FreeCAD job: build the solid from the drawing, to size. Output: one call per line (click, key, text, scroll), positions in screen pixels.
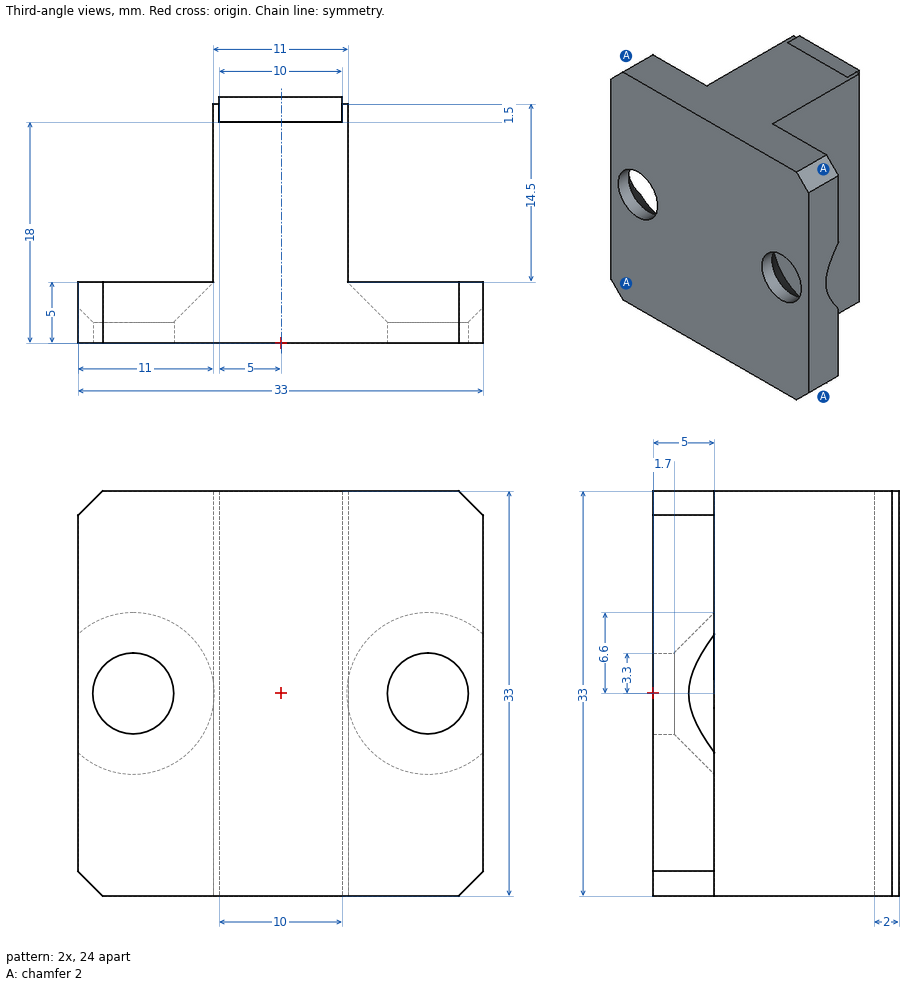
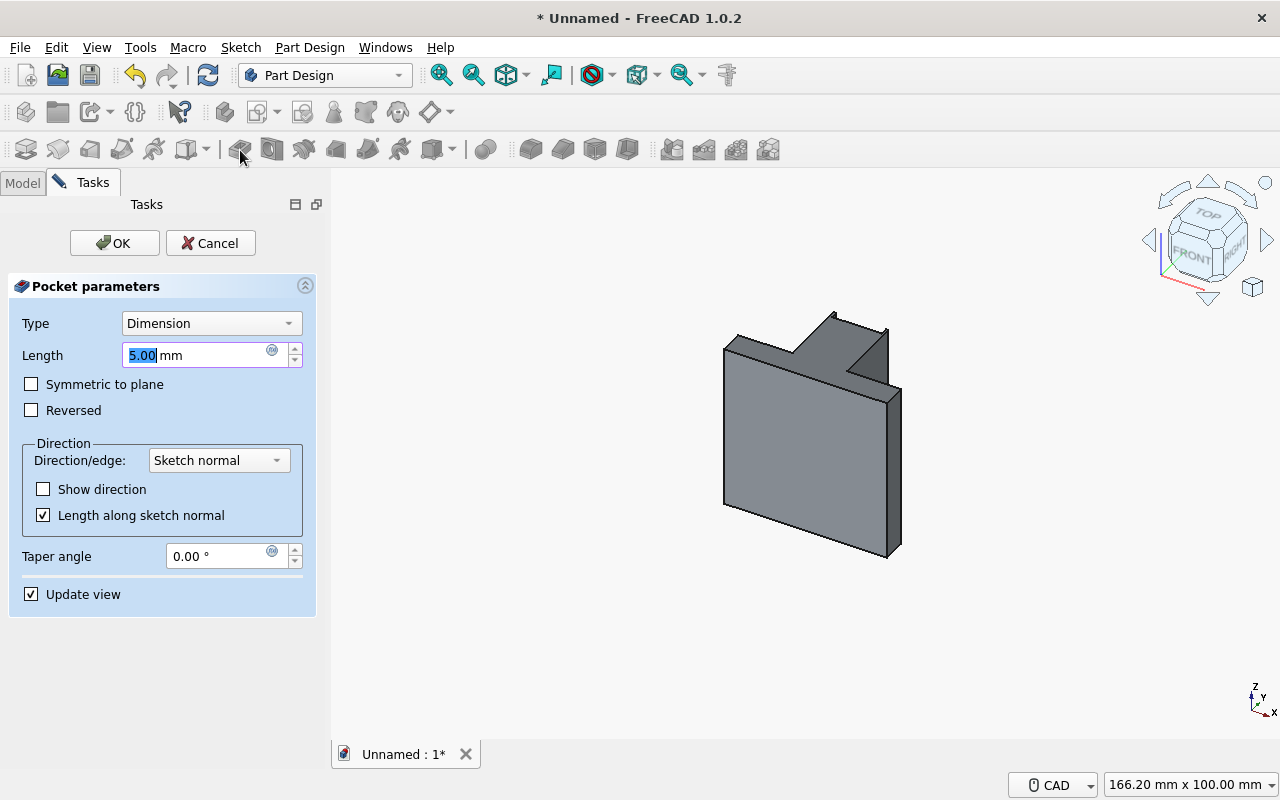
click(212, 324)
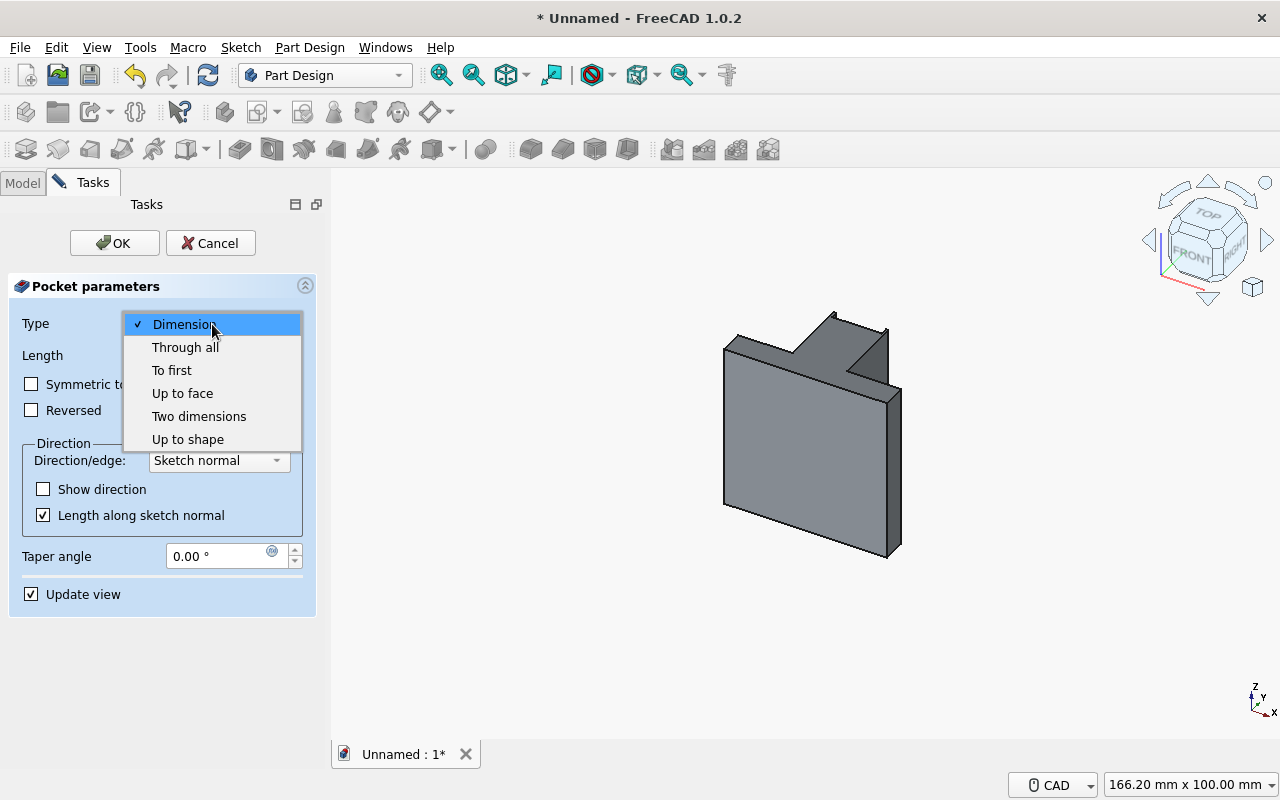
click(212, 348)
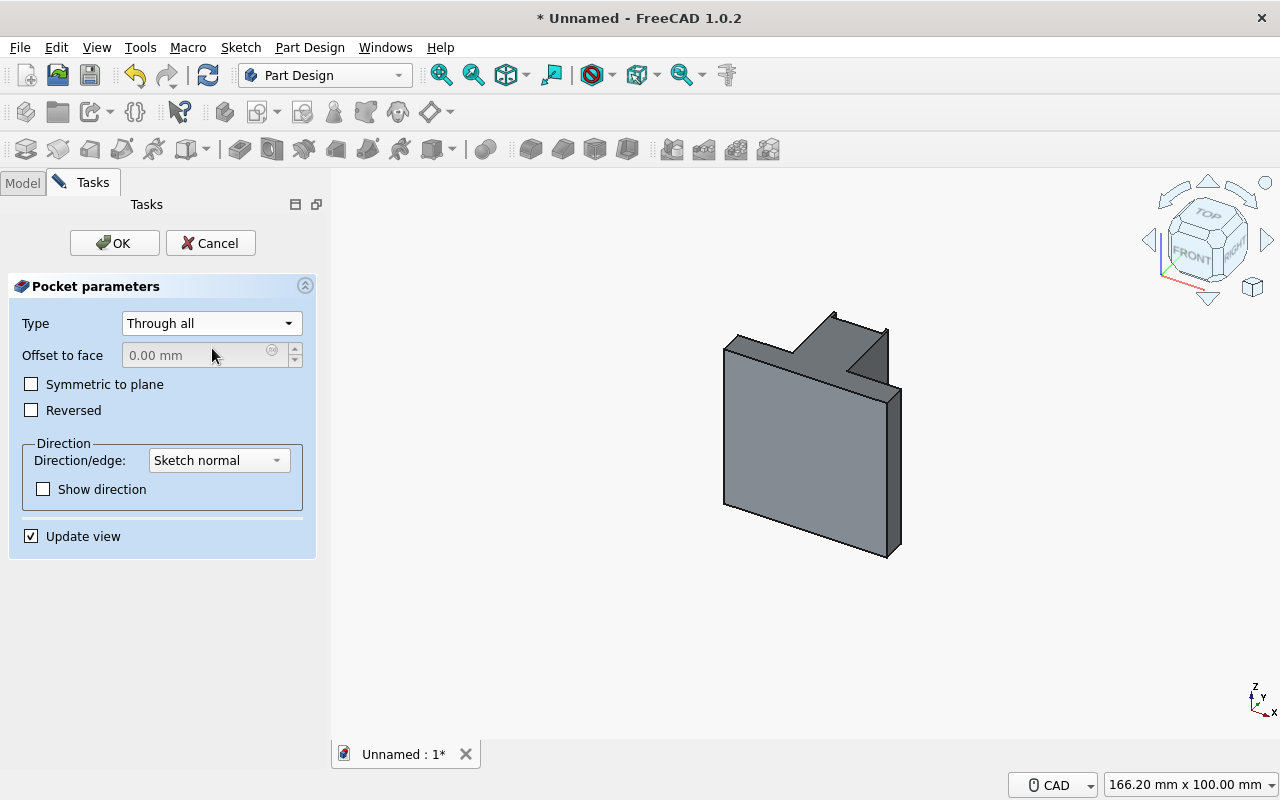
click(115, 243)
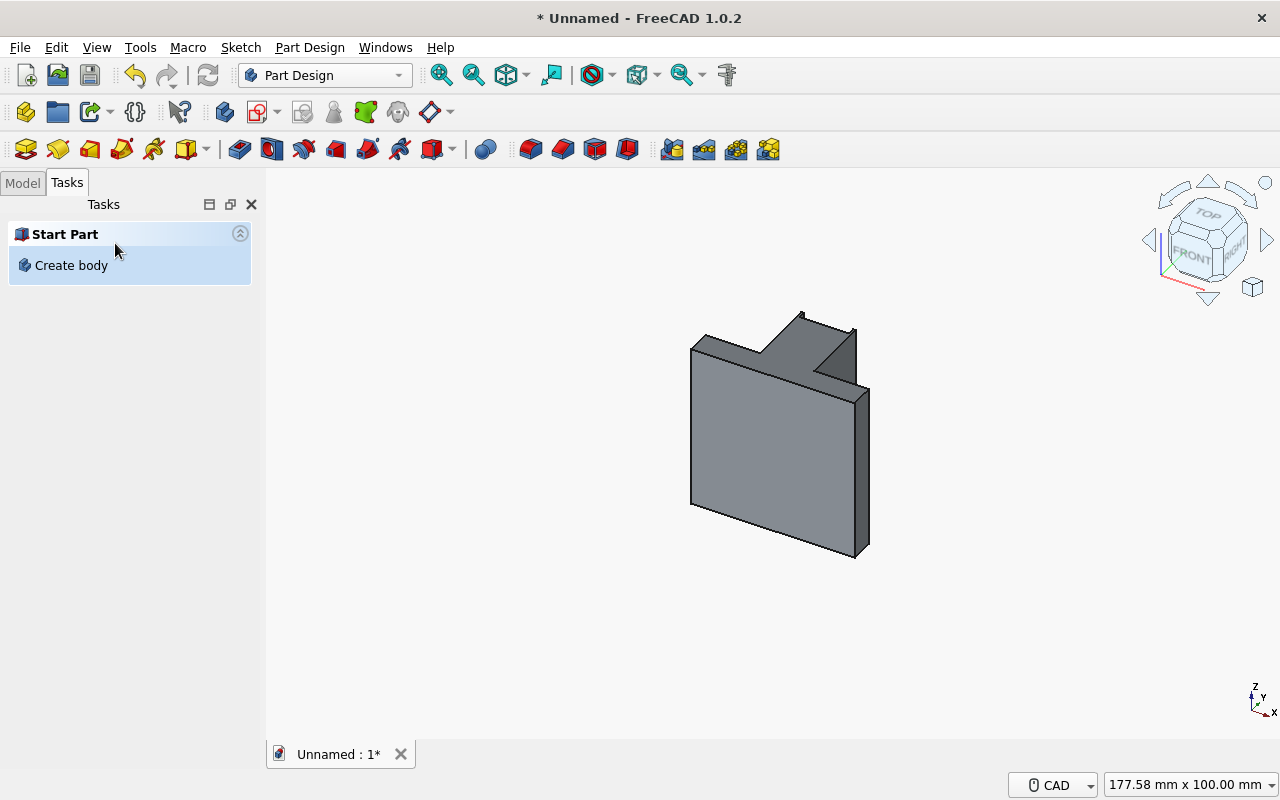
click(23, 182)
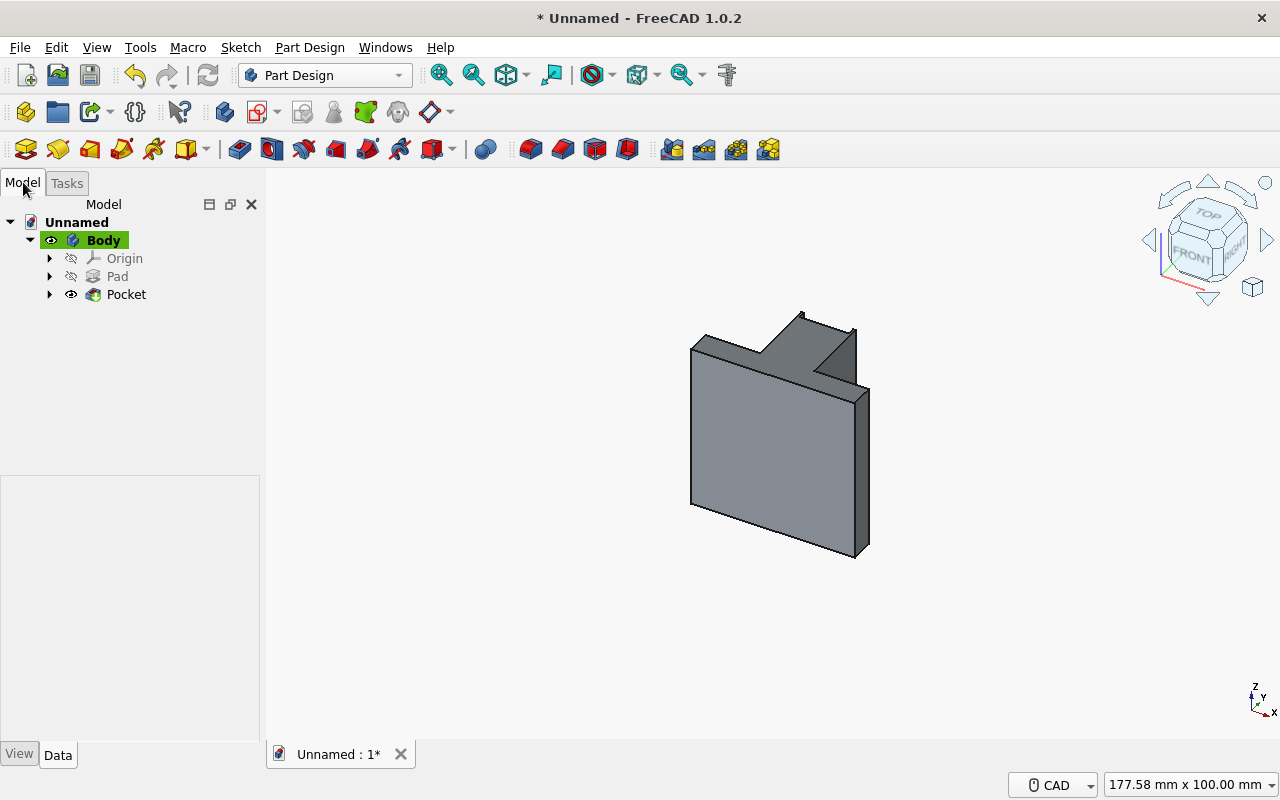
click(50, 258)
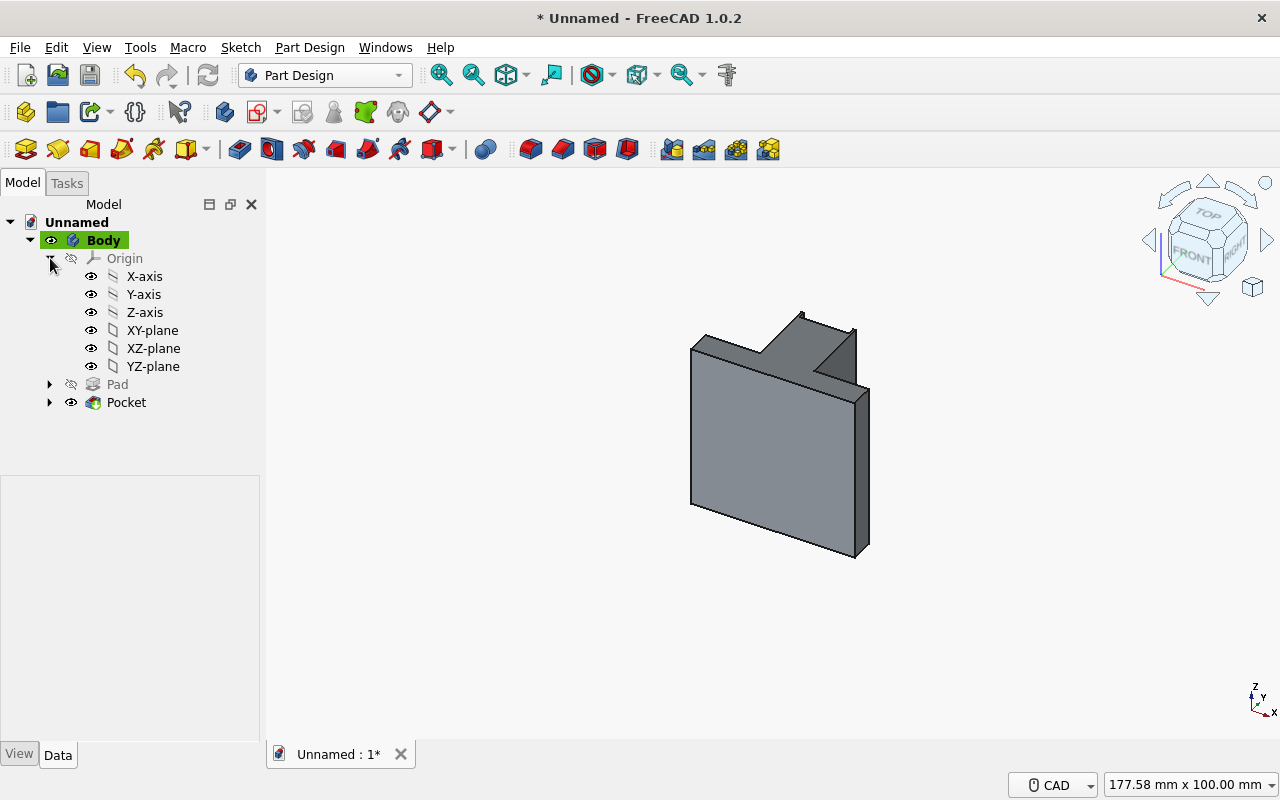
click(136, 366)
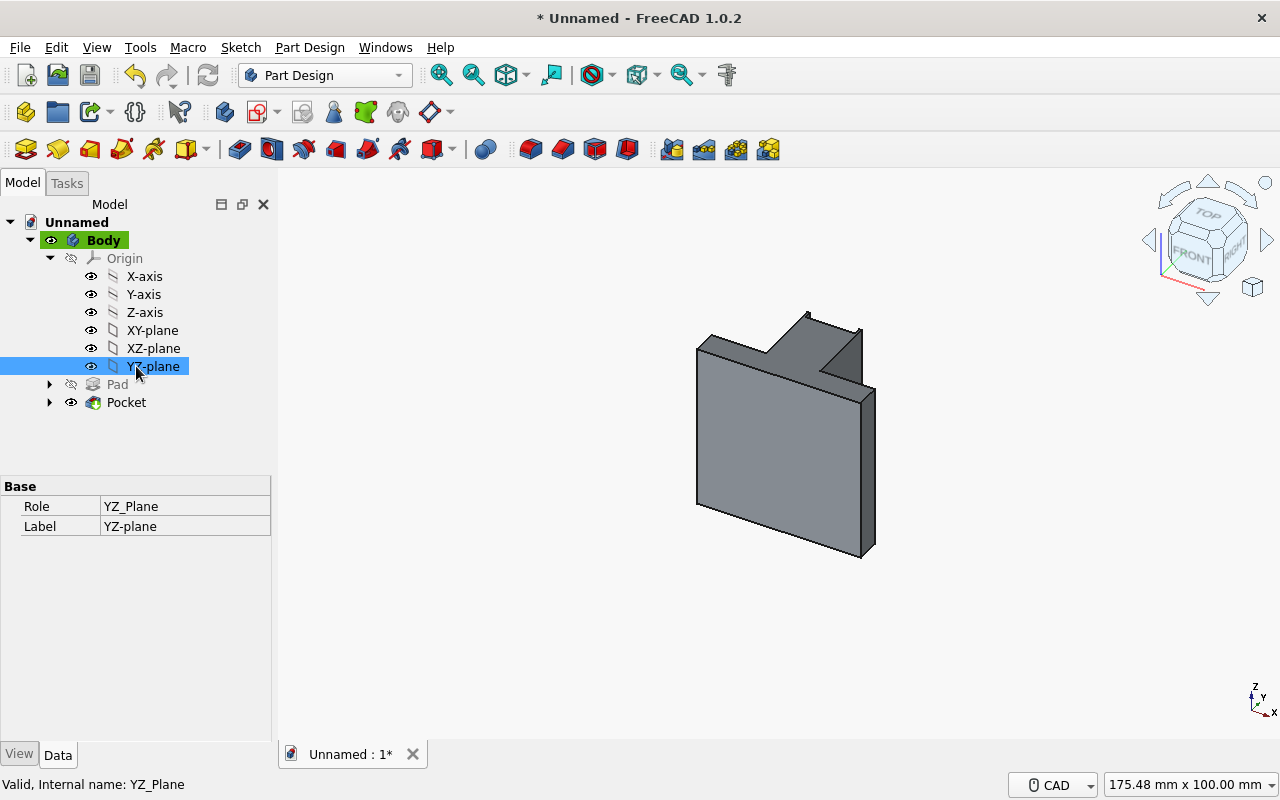
click(430, 112)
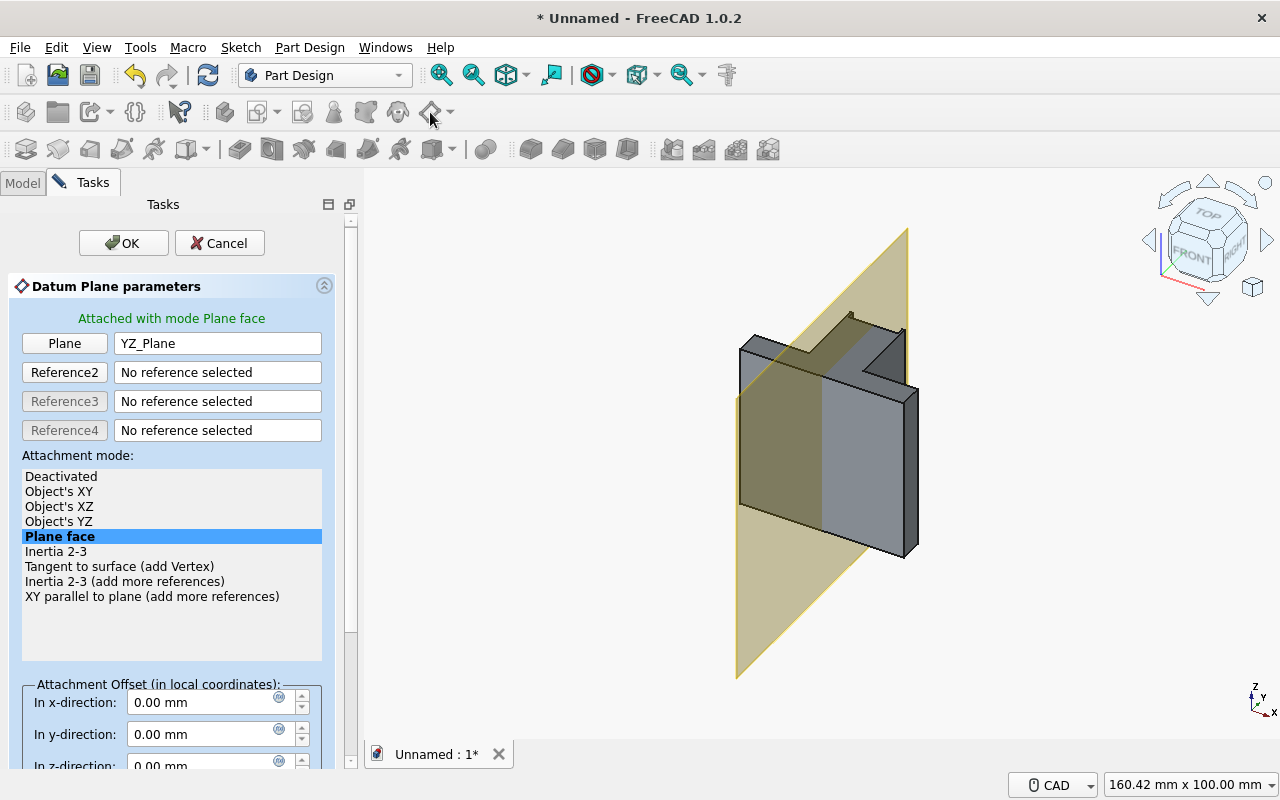
scroll(351, 491, down, 2)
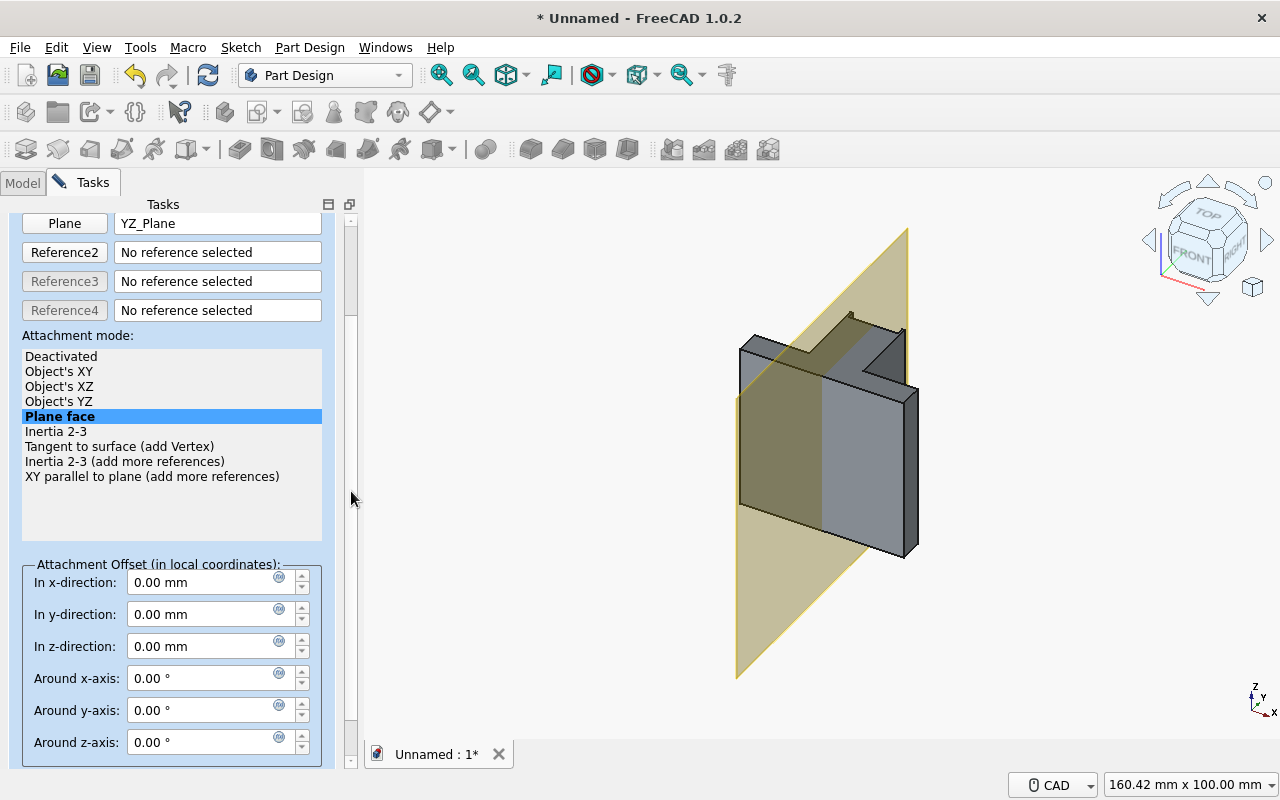
triple_click(210, 646)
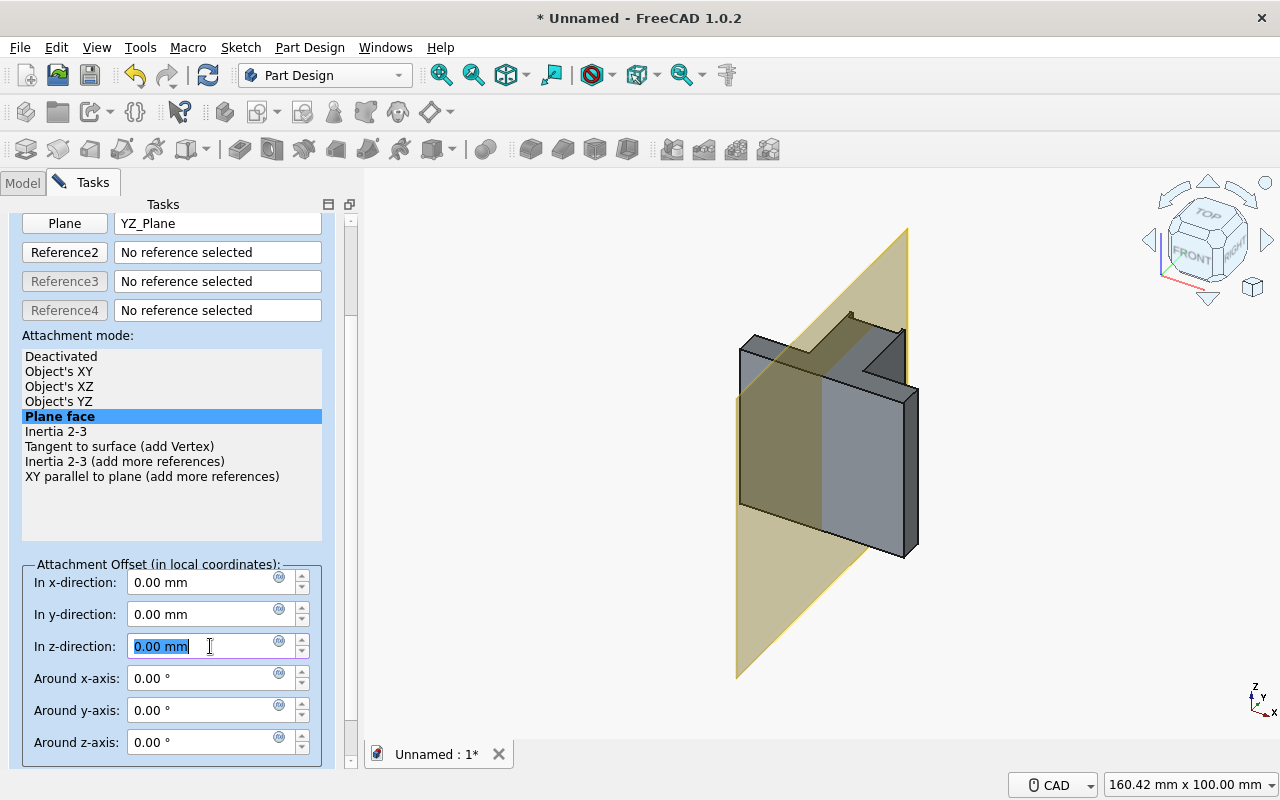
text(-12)
key(Tab)